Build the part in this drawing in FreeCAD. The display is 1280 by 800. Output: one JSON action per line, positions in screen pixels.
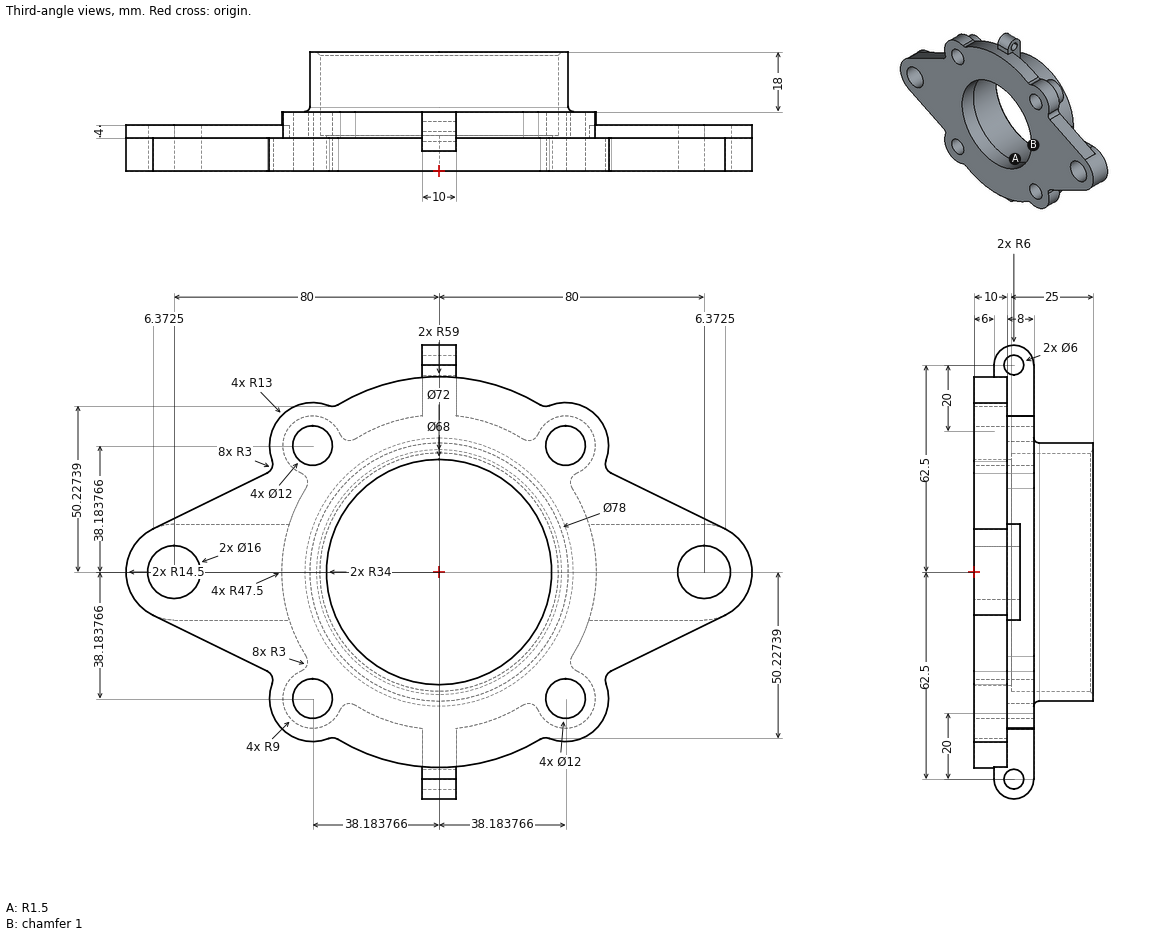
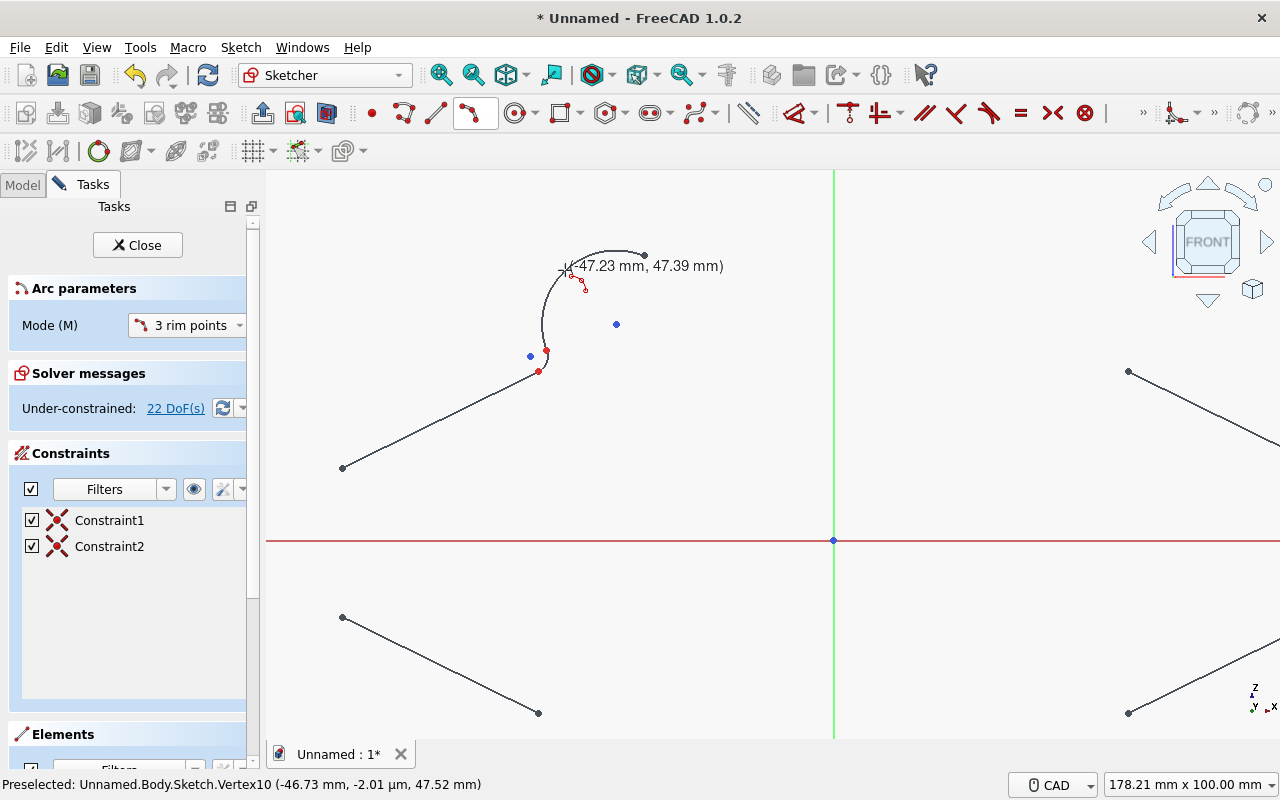
{"action": "left_click", "coordinate": [644, 256]}
{"action": "left_click", "coordinate": [660, 254]}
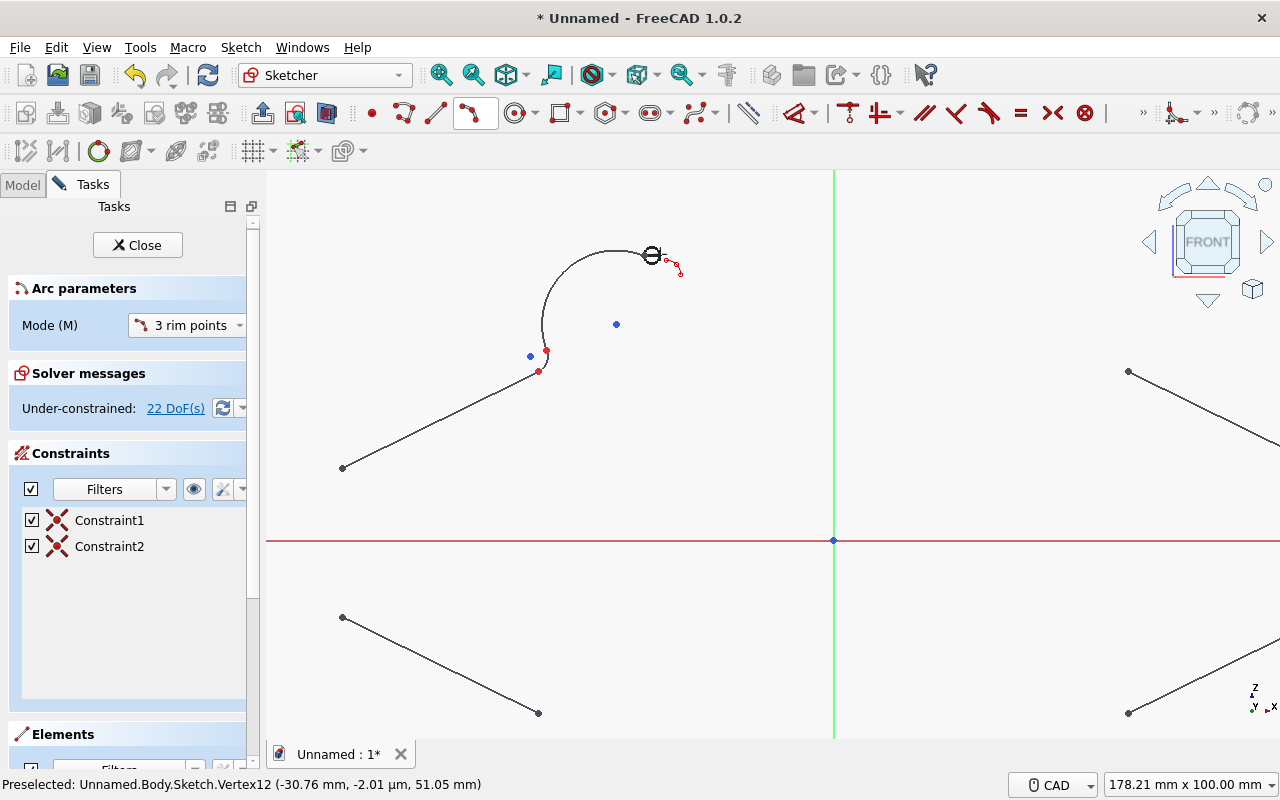
{"action": "scroll", "coordinate": [652, 256], "scroll_direction": "up", "scroll_amount": 11}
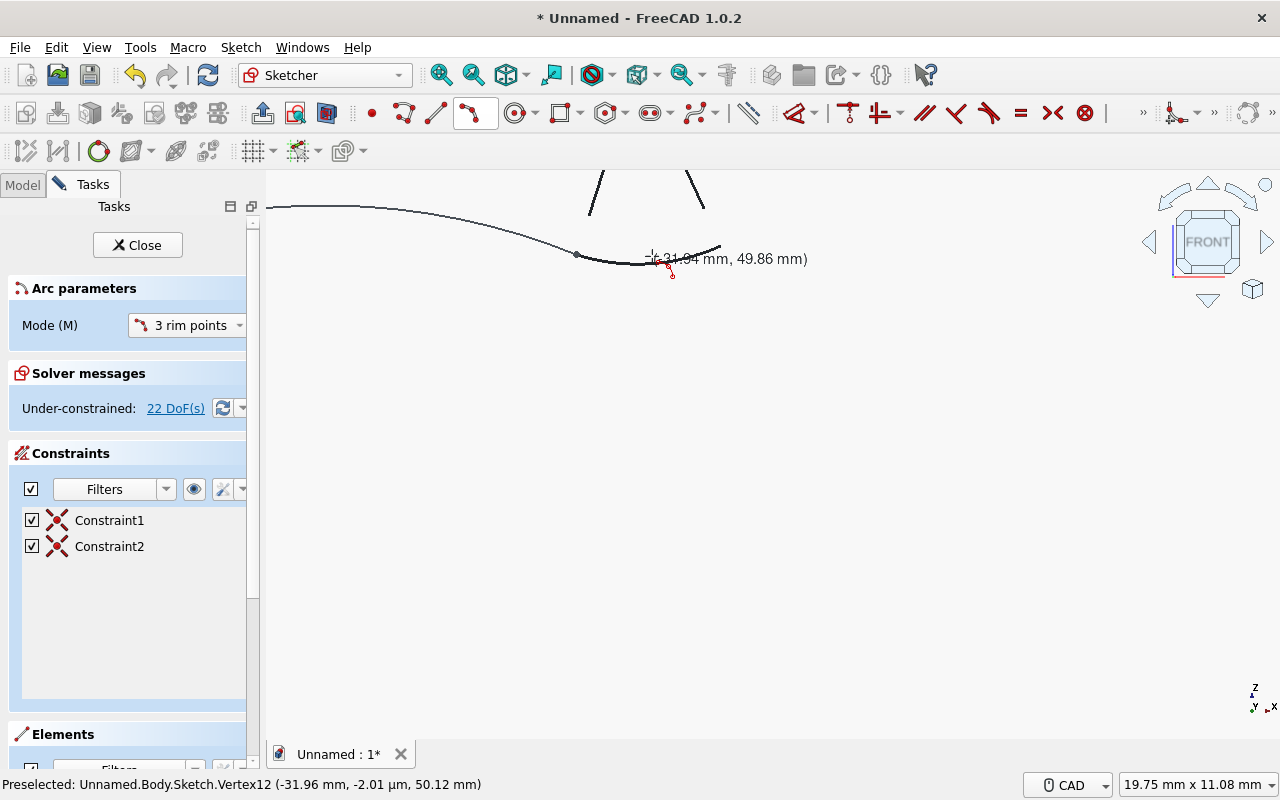
{"action": "left_click", "coordinate": [650, 256]}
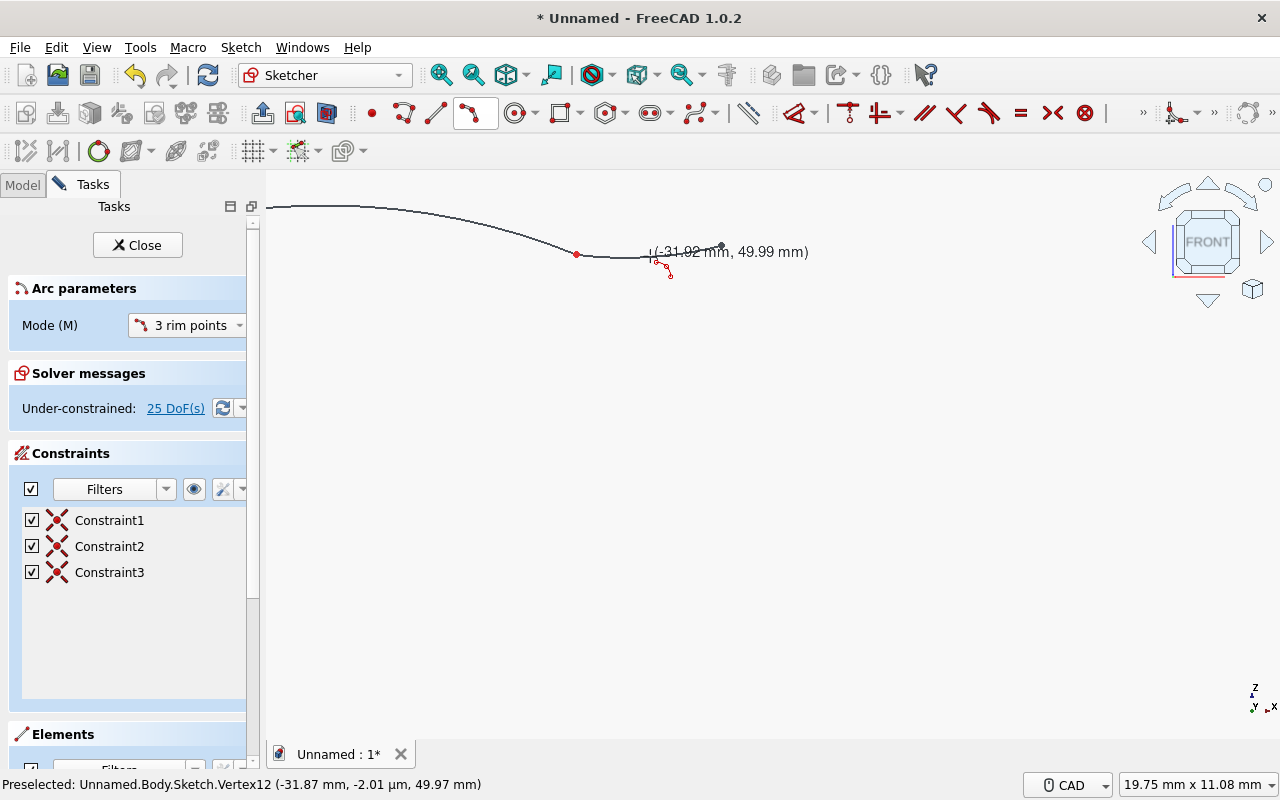
{"action": "scroll", "coordinate": [602, 301], "scroll_direction": "down", "scroll_amount": 14}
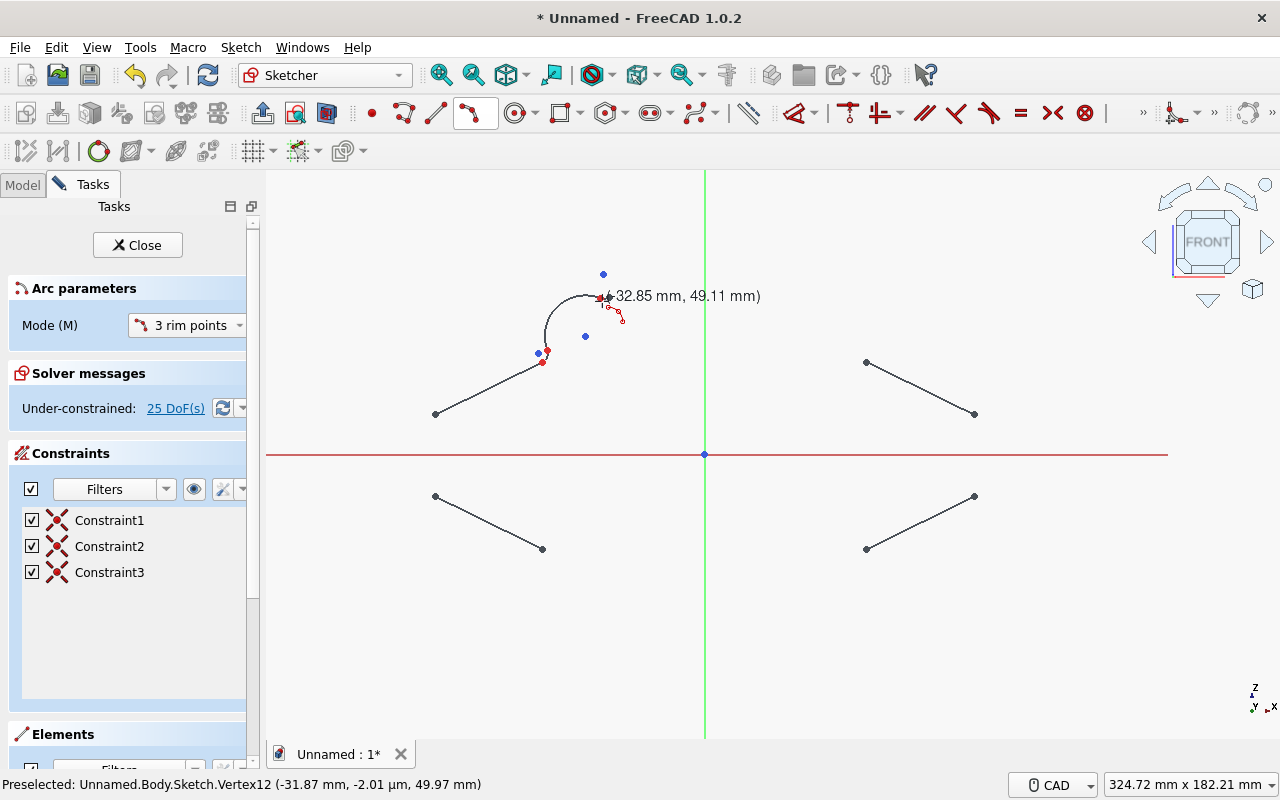
{"action": "scroll", "coordinate": [609, 297], "scroll_direction": "up", "scroll_amount": 4}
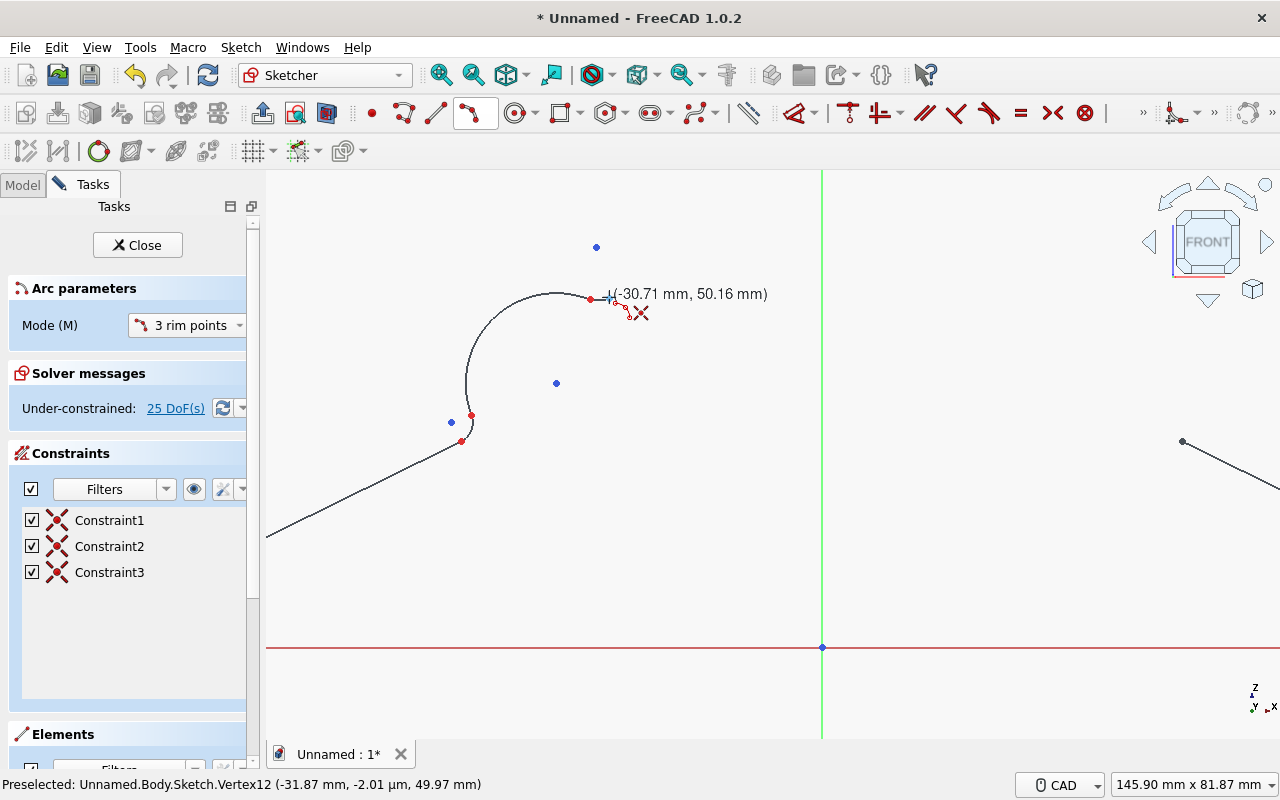
{"action": "left_click", "coordinate": [610, 299]}
{"action": "left_click", "coordinate": [1035, 297]}
{"action": "left_click", "coordinate": [867, 240]}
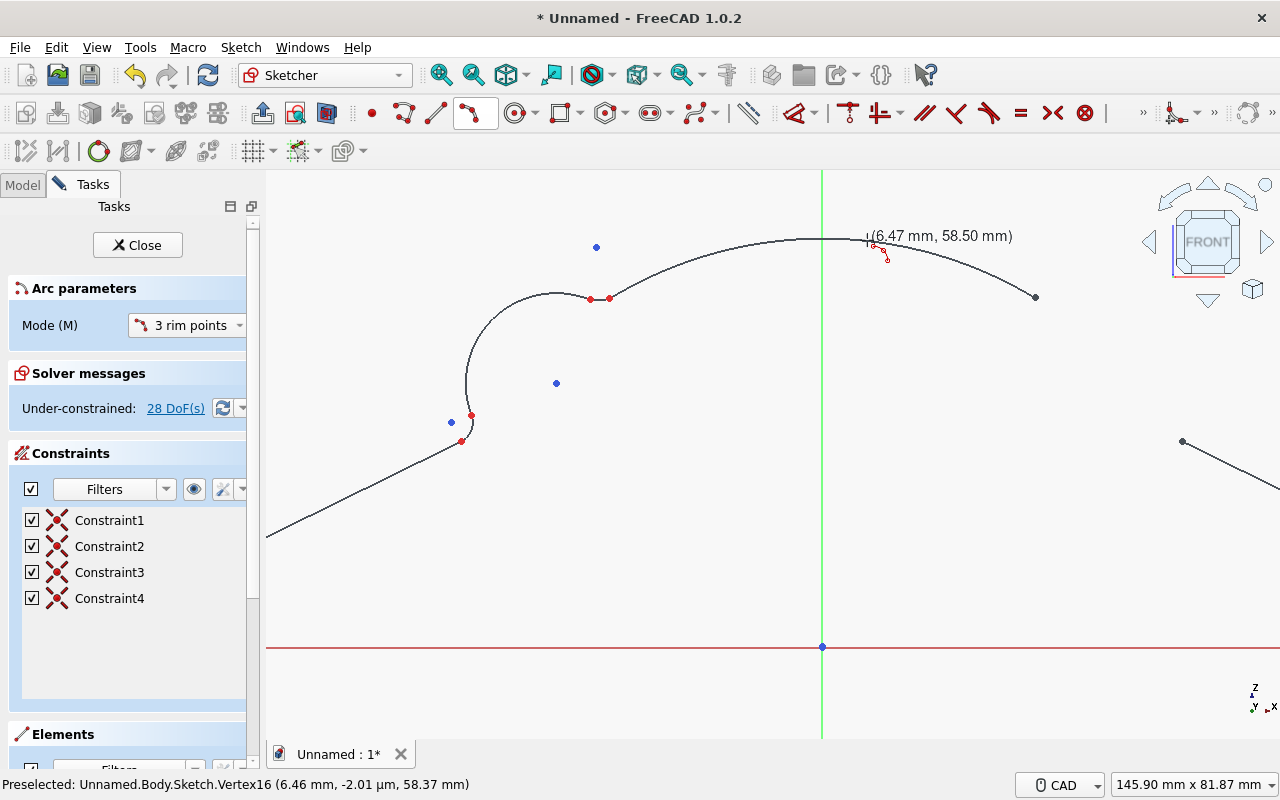
{"action": "left_click", "coordinate": [1035, 298]}
{"action": "left_click", "coordinate": [1053, 298]}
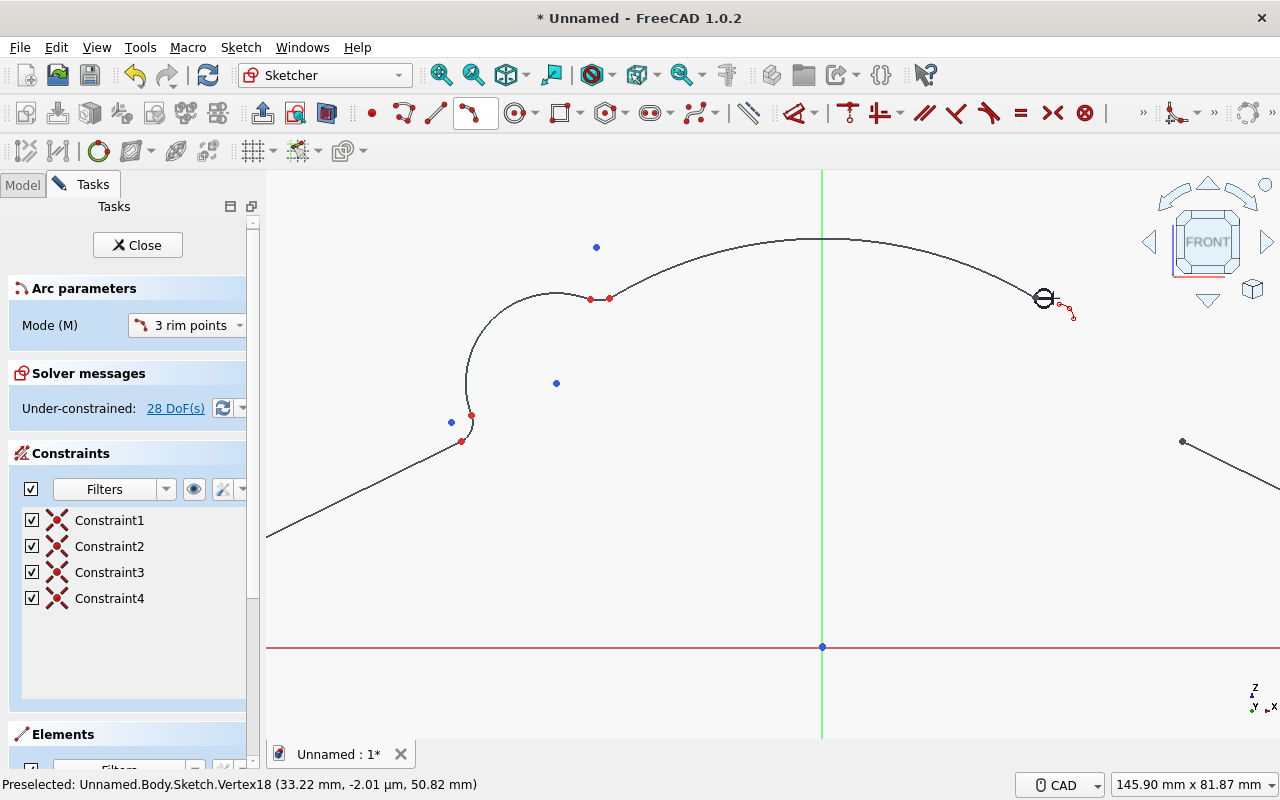
{"action": "scroll", "coordinate": [1044, 300], "scroll_direction": "up", "scroll_amount": 10}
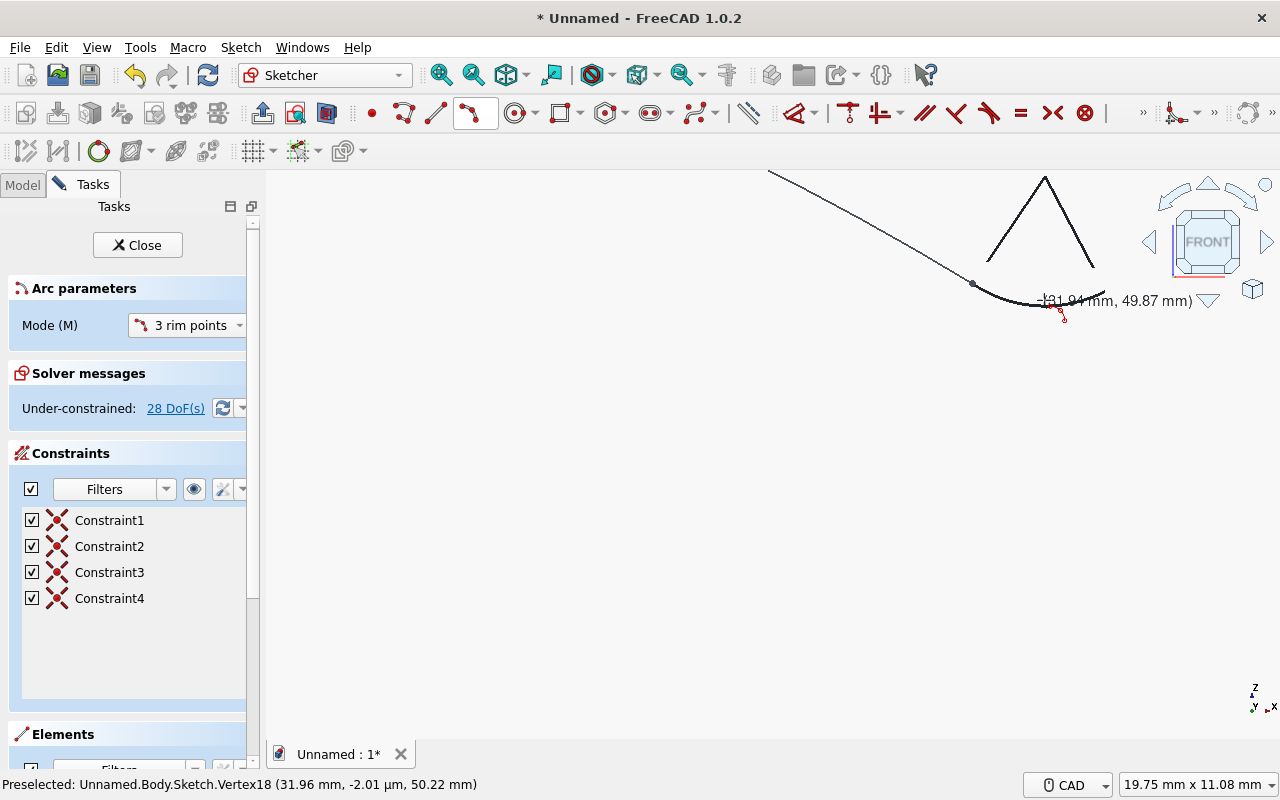
{"action": "left_click", "coordinate": [1038, 298]}